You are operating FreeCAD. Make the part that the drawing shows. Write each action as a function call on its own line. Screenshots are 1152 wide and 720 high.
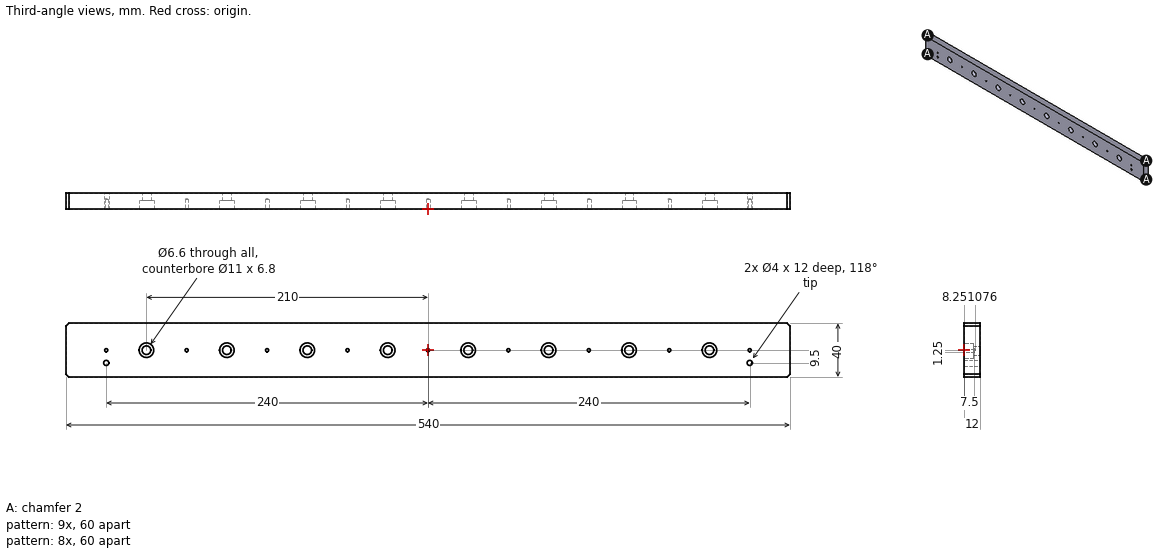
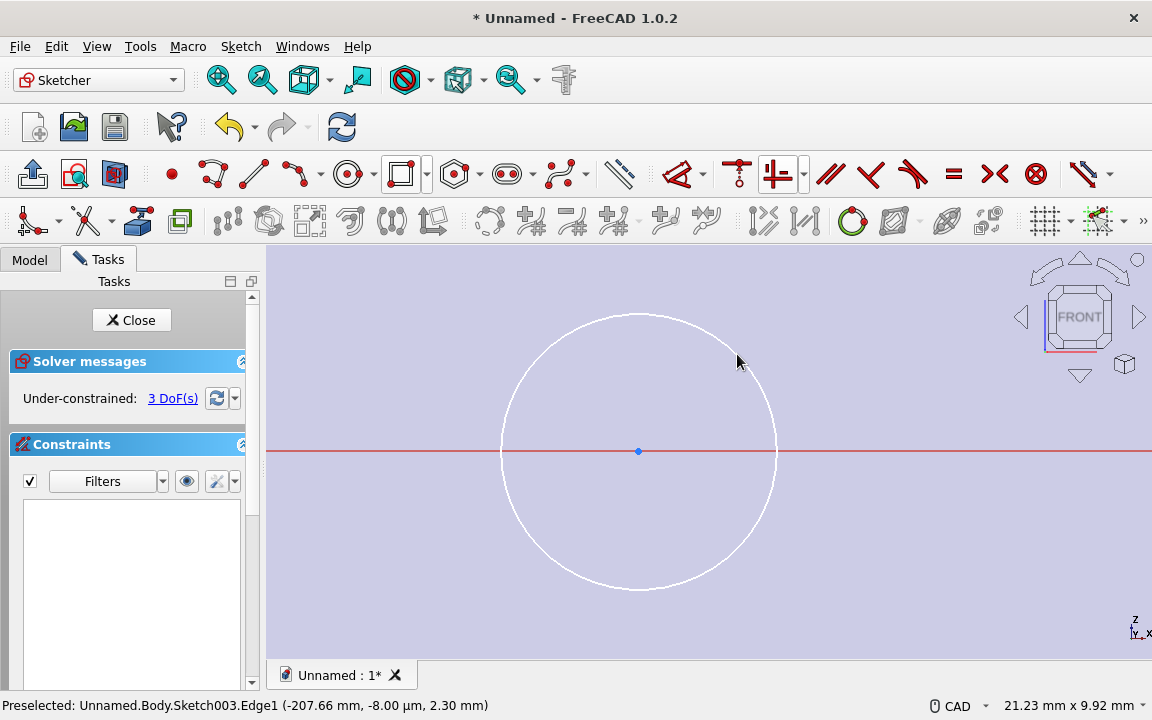
click(639, 452)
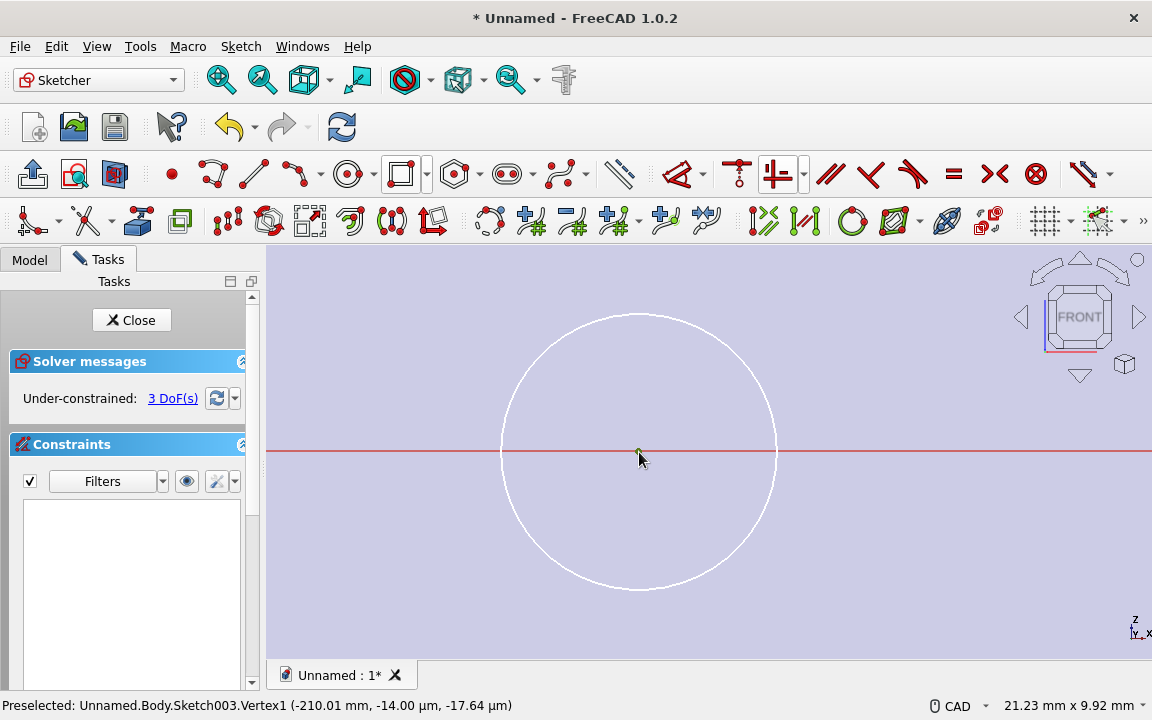
click(344, 451)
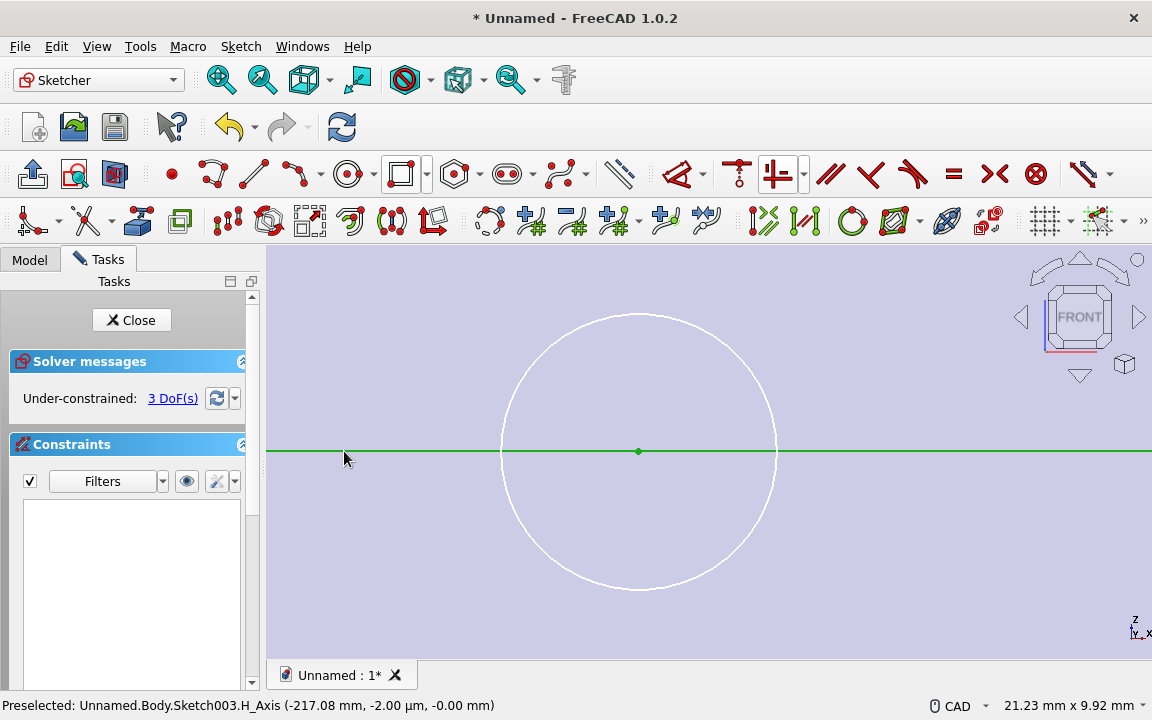
key(c)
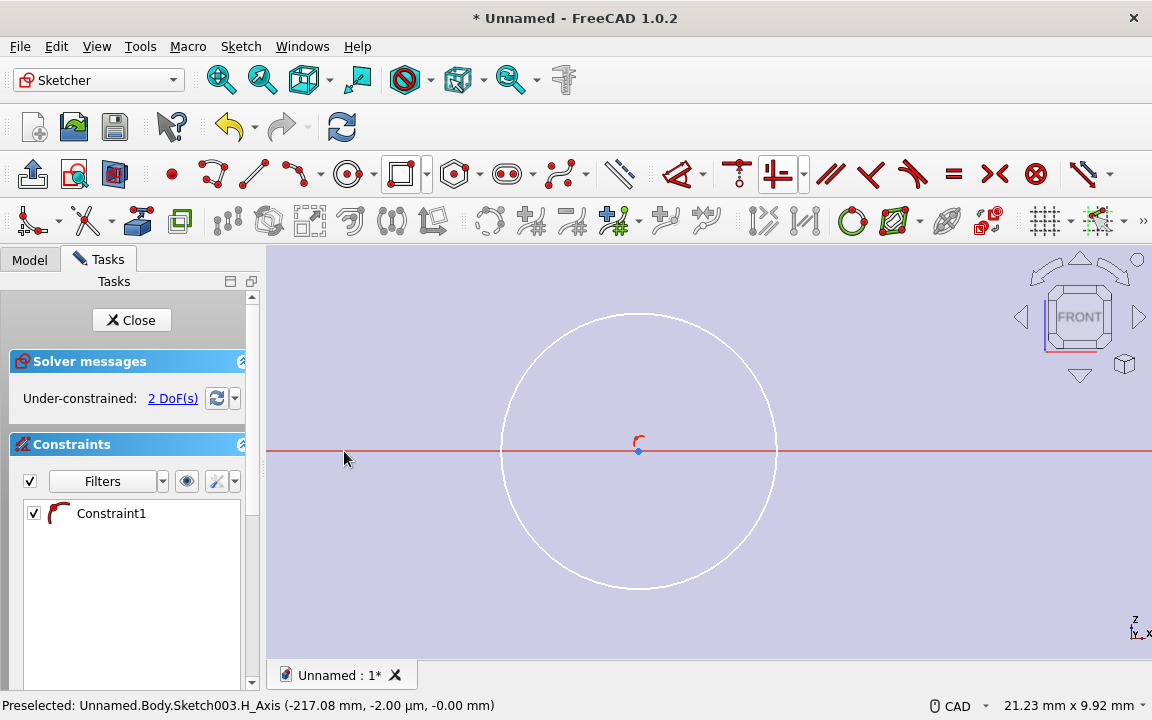
click(676, 174)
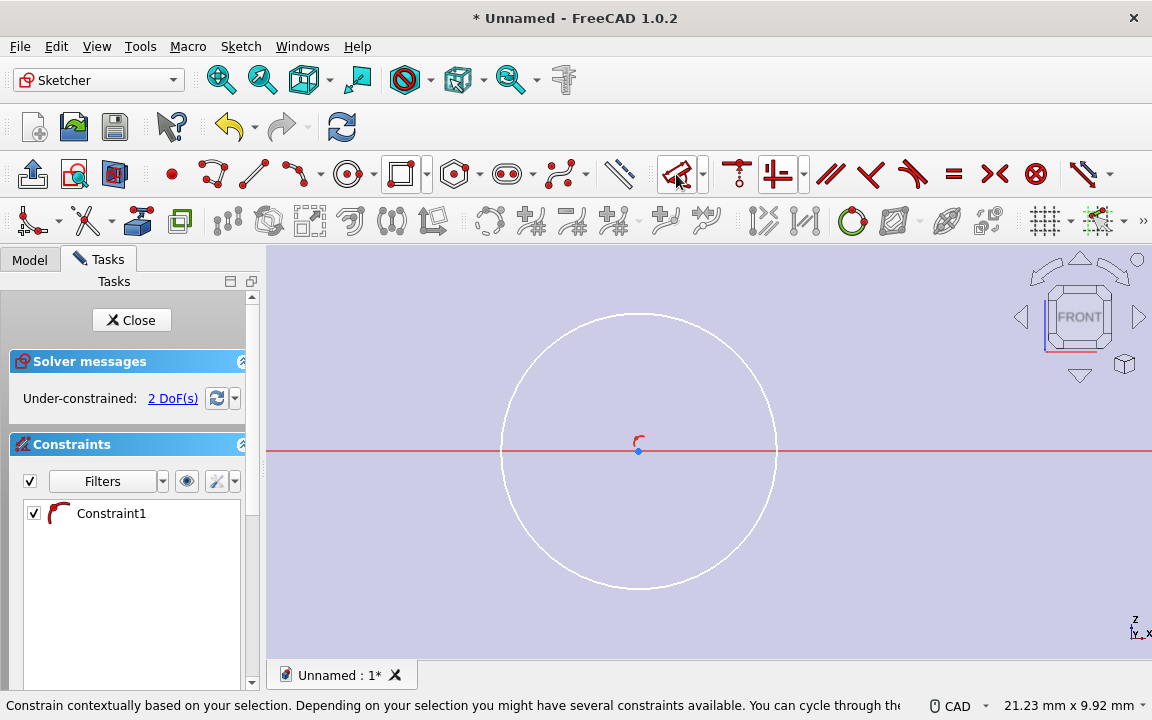
click(736, 353)
click(758, 330)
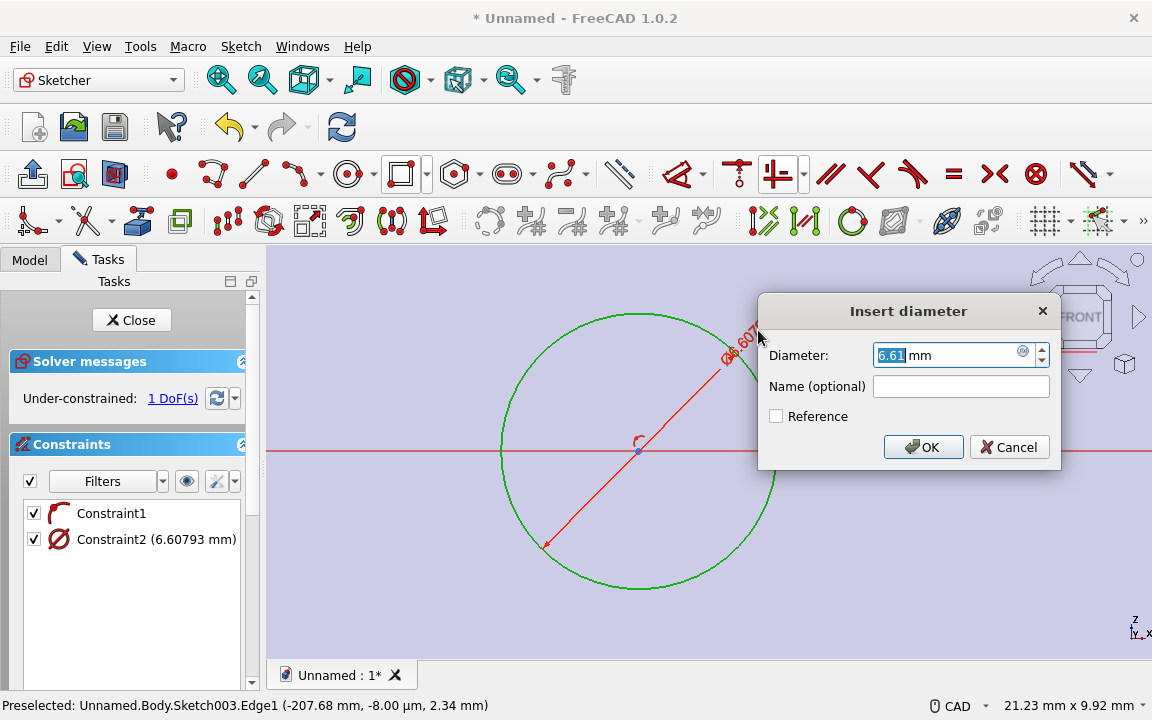
text(6.6)
key(Return)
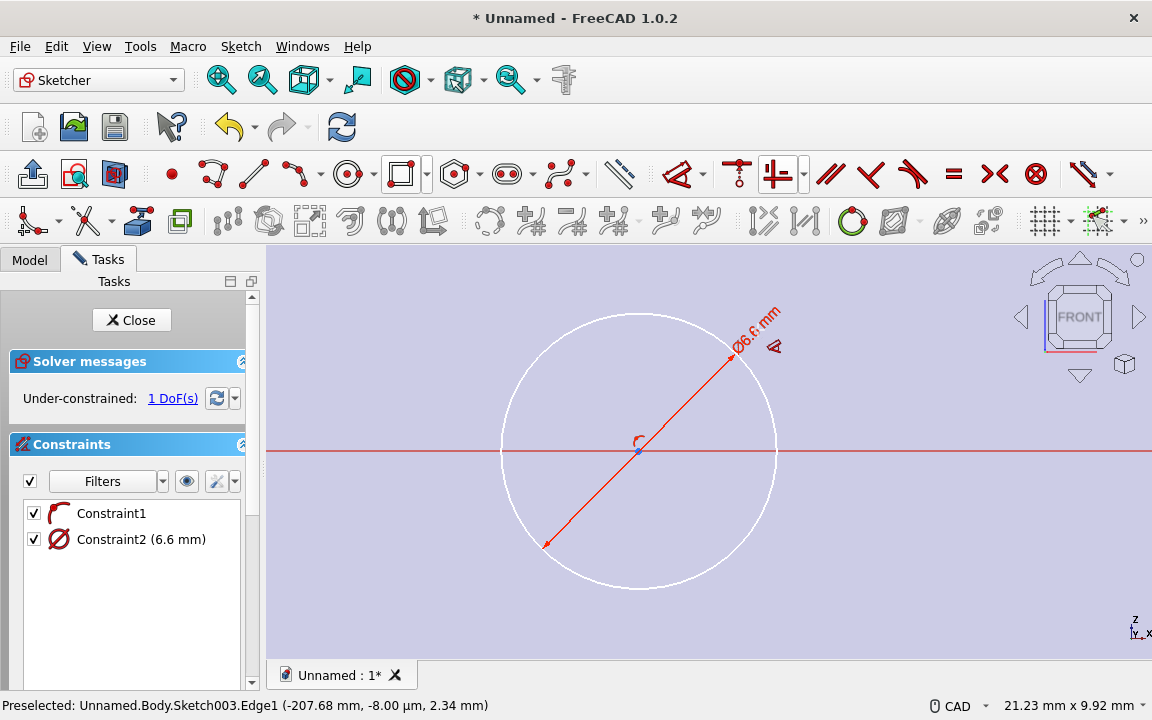
click(639, 451)
click(813, 485)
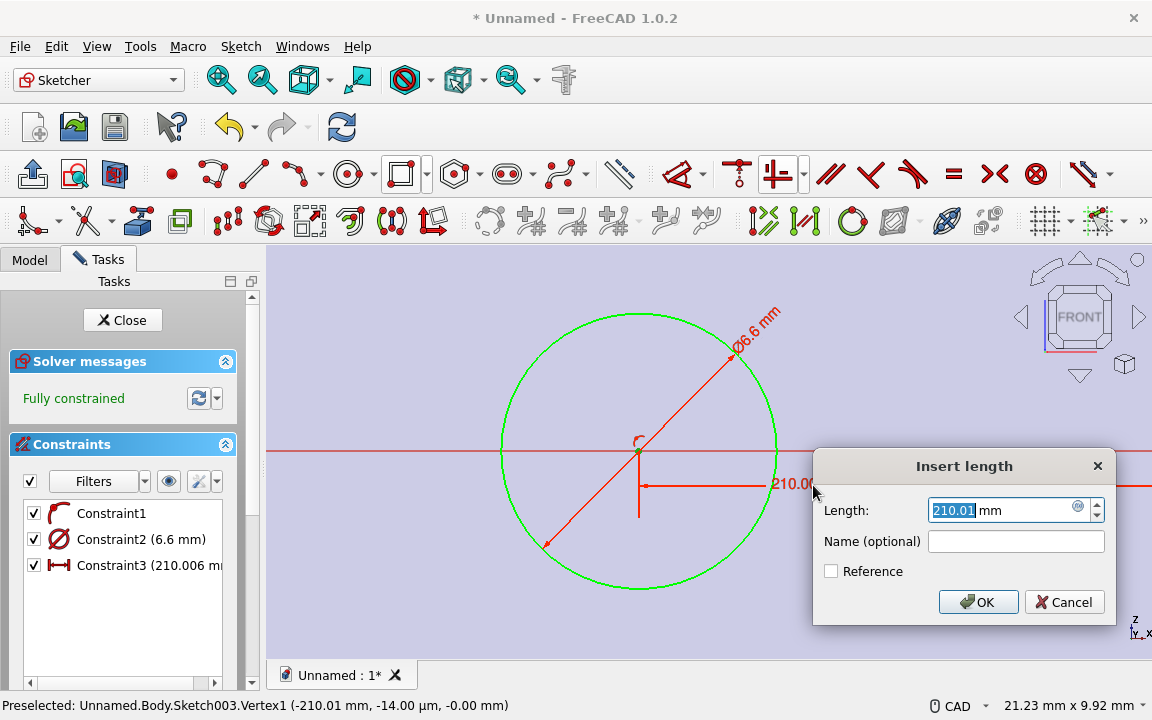
text(210)
key(Return)
key(Escape)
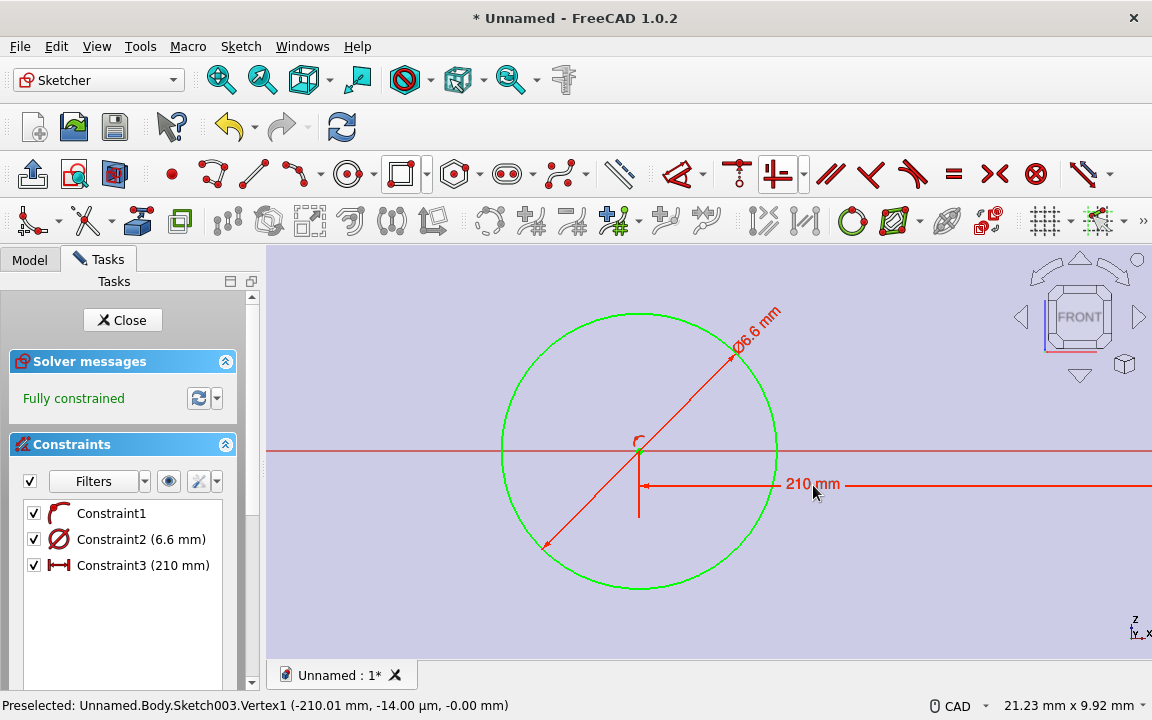
click(123, 320)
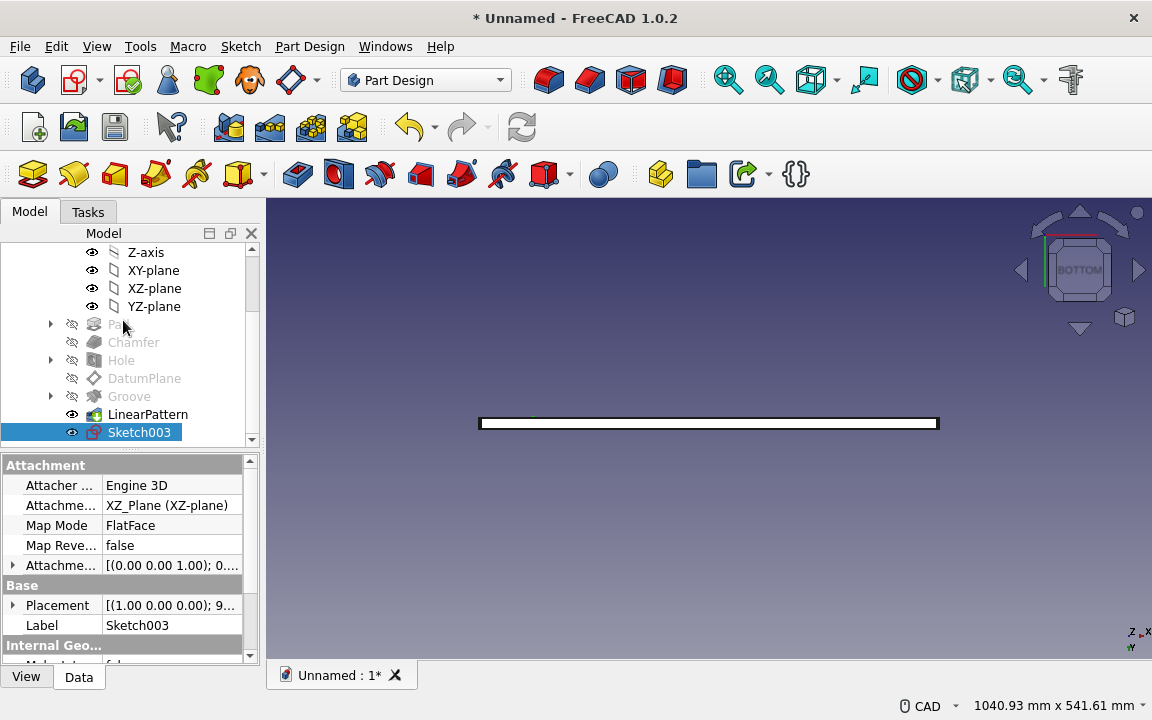
click(339, 174)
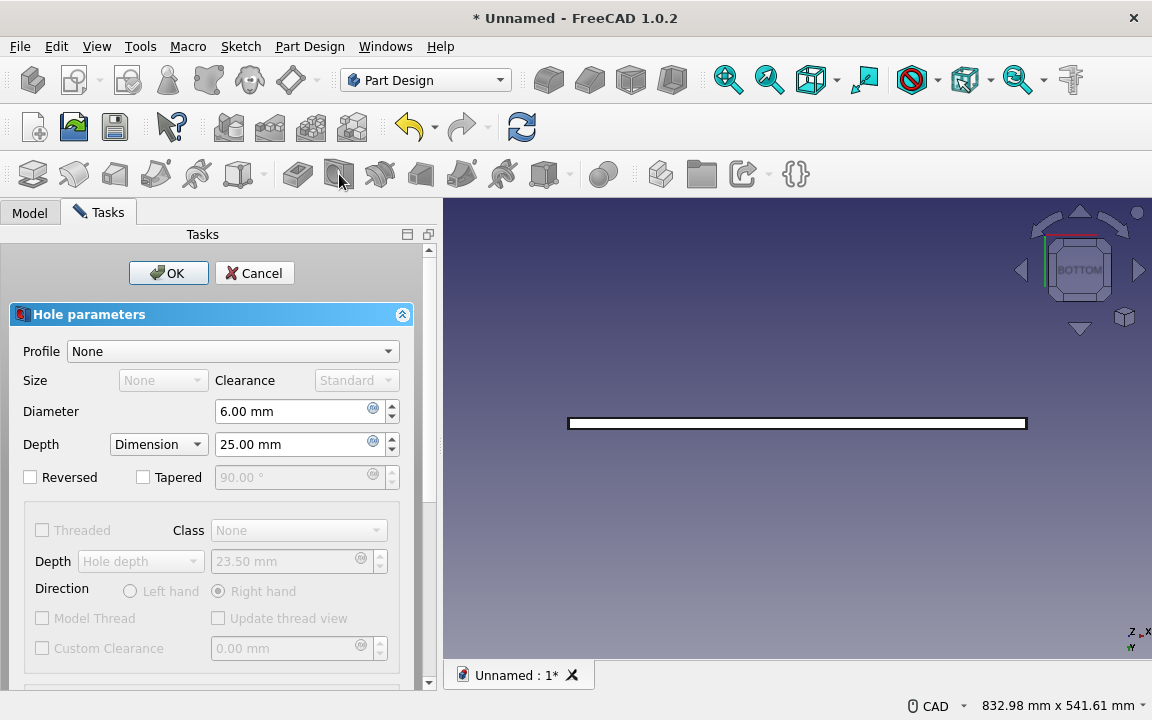
triple_click(300, 412)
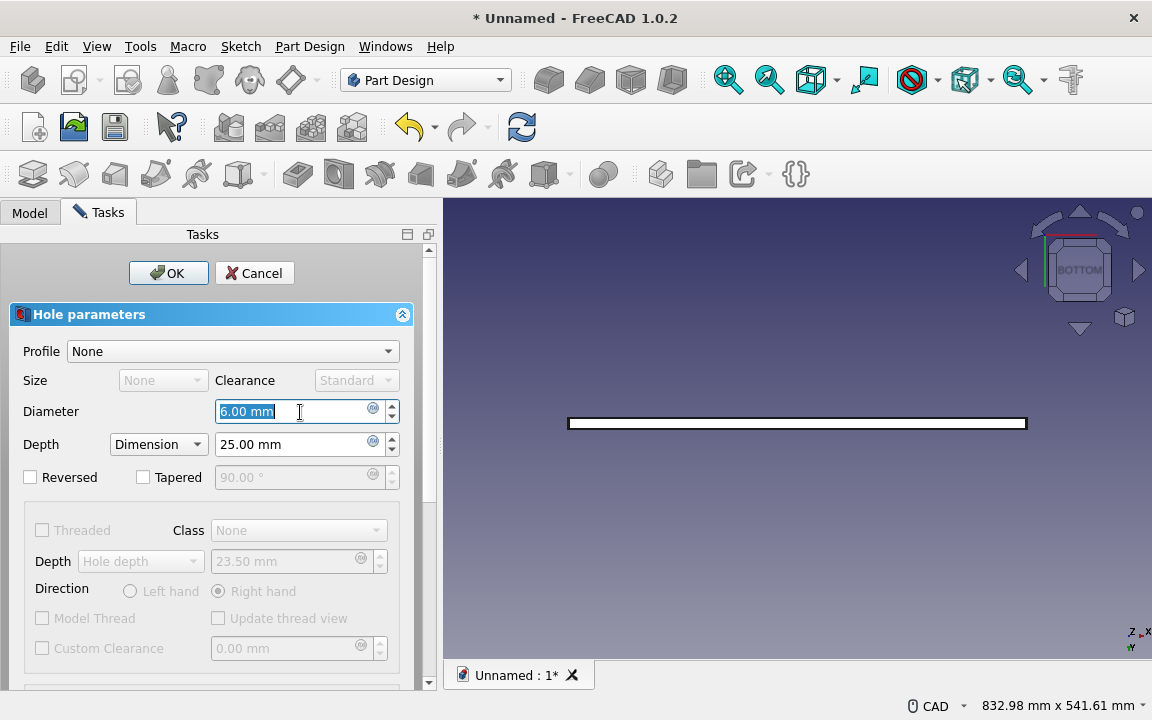
text(6.6)
key(Tab)